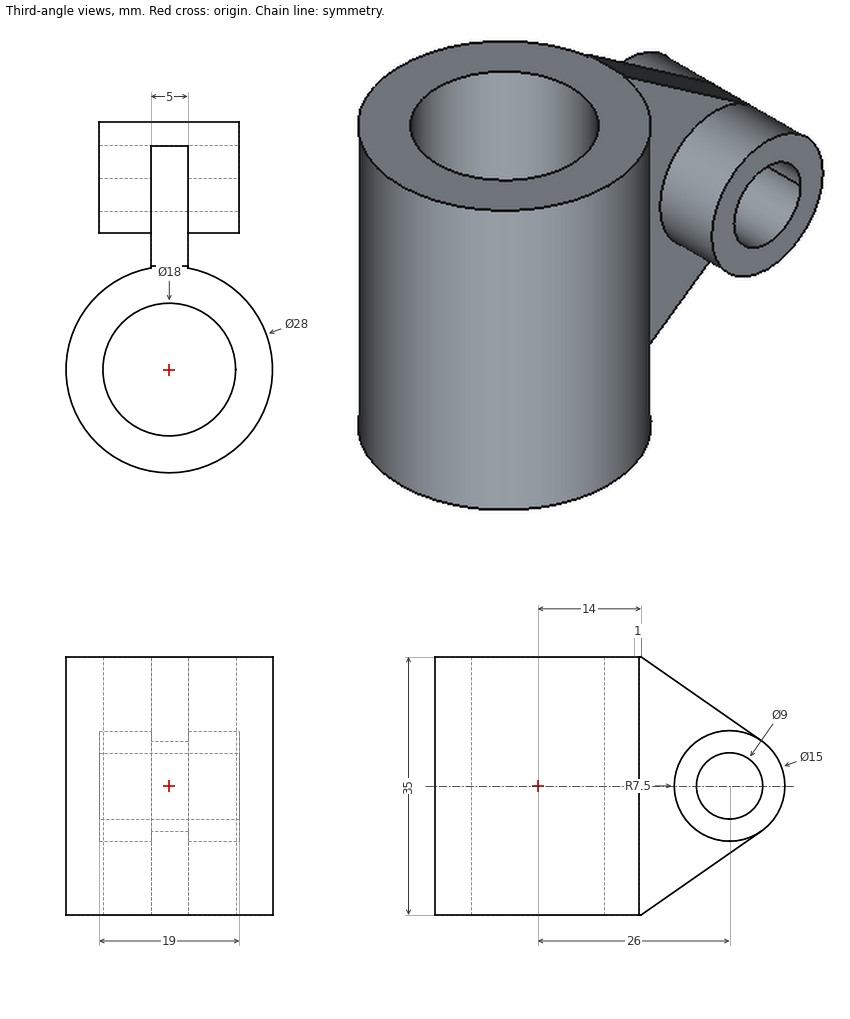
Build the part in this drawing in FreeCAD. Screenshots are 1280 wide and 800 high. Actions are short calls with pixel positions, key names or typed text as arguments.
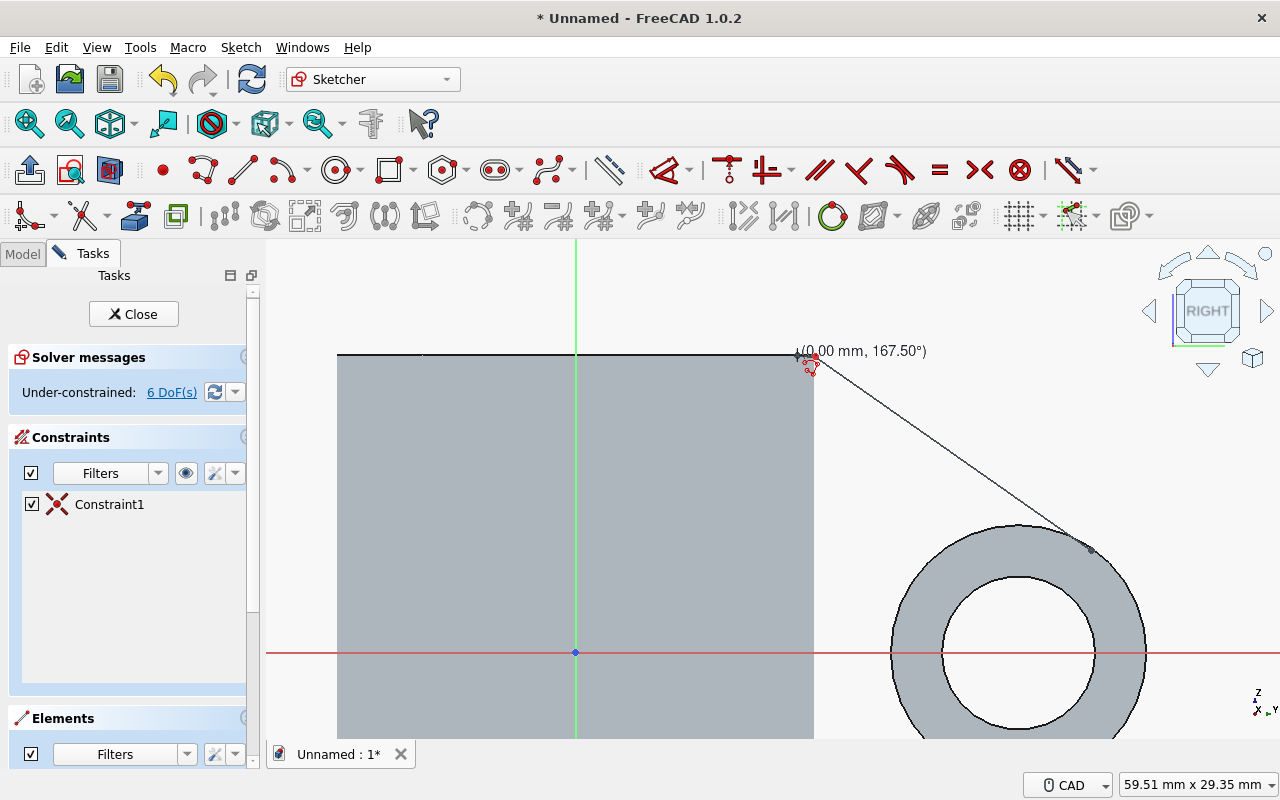
scroll(547, 290, down, 3)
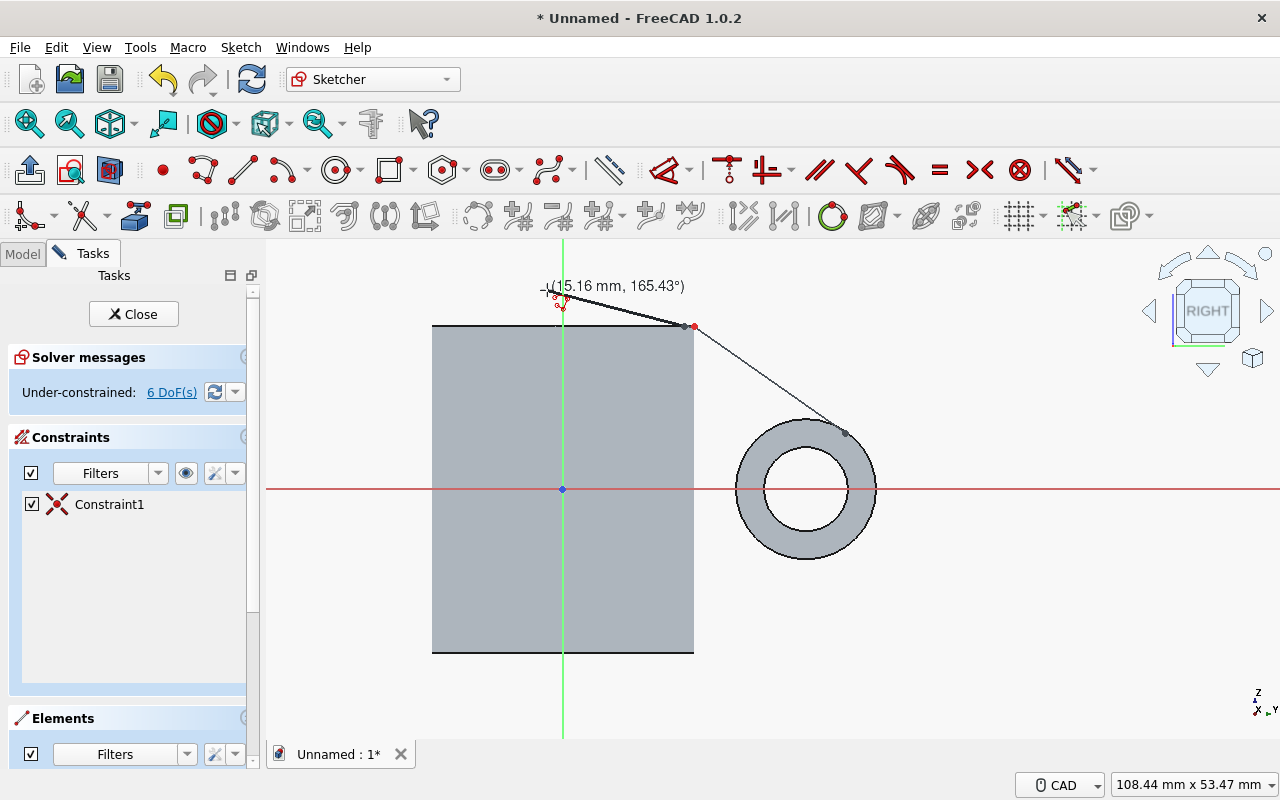
click(684, 653)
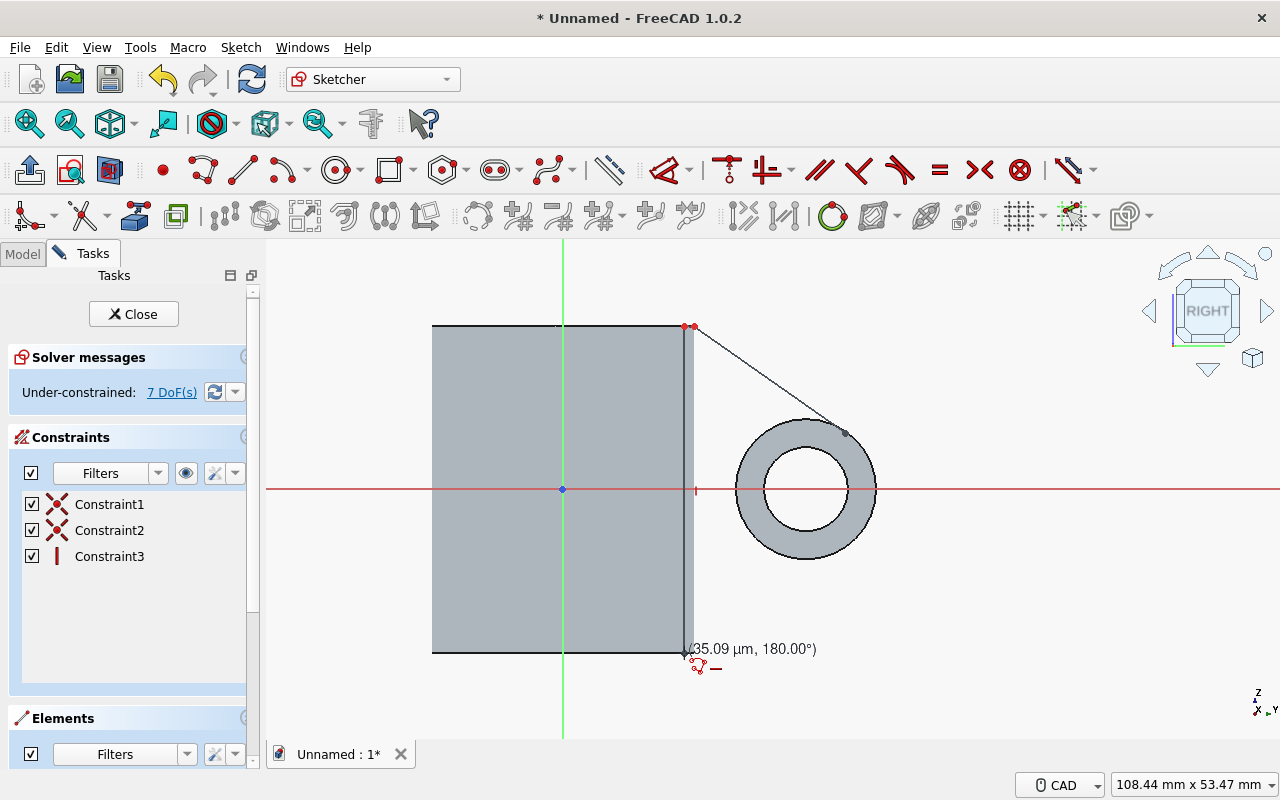
scroll(694, 653, up, 3)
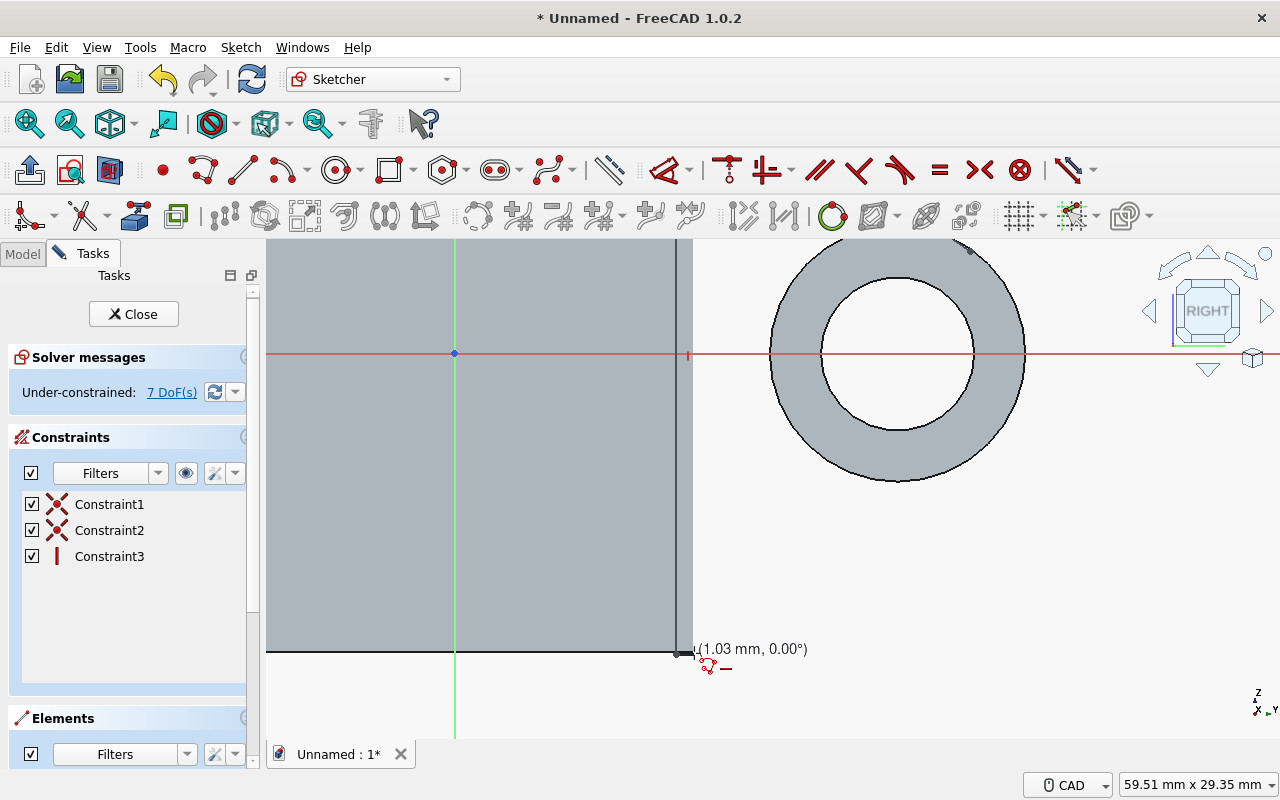
click(693, 652)
click(971, 459)
right_click(971, 459)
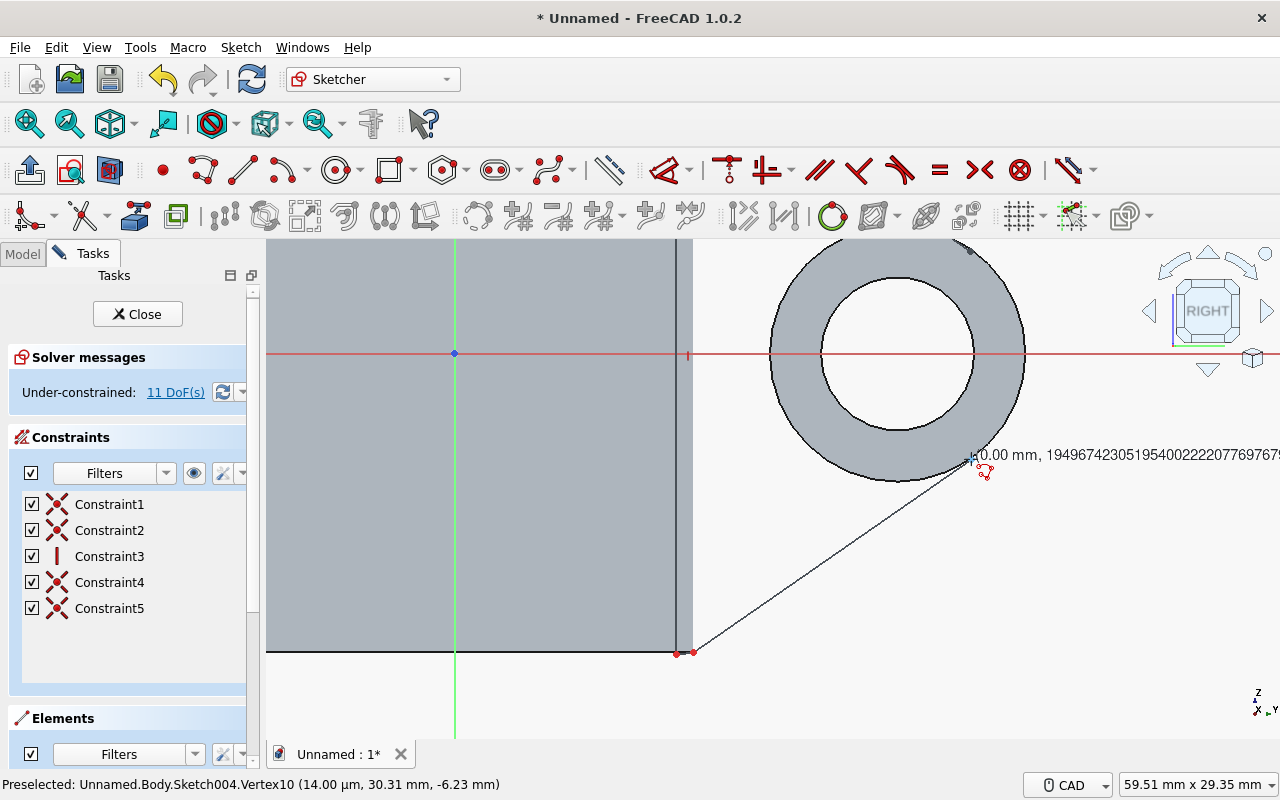
click(310, 170)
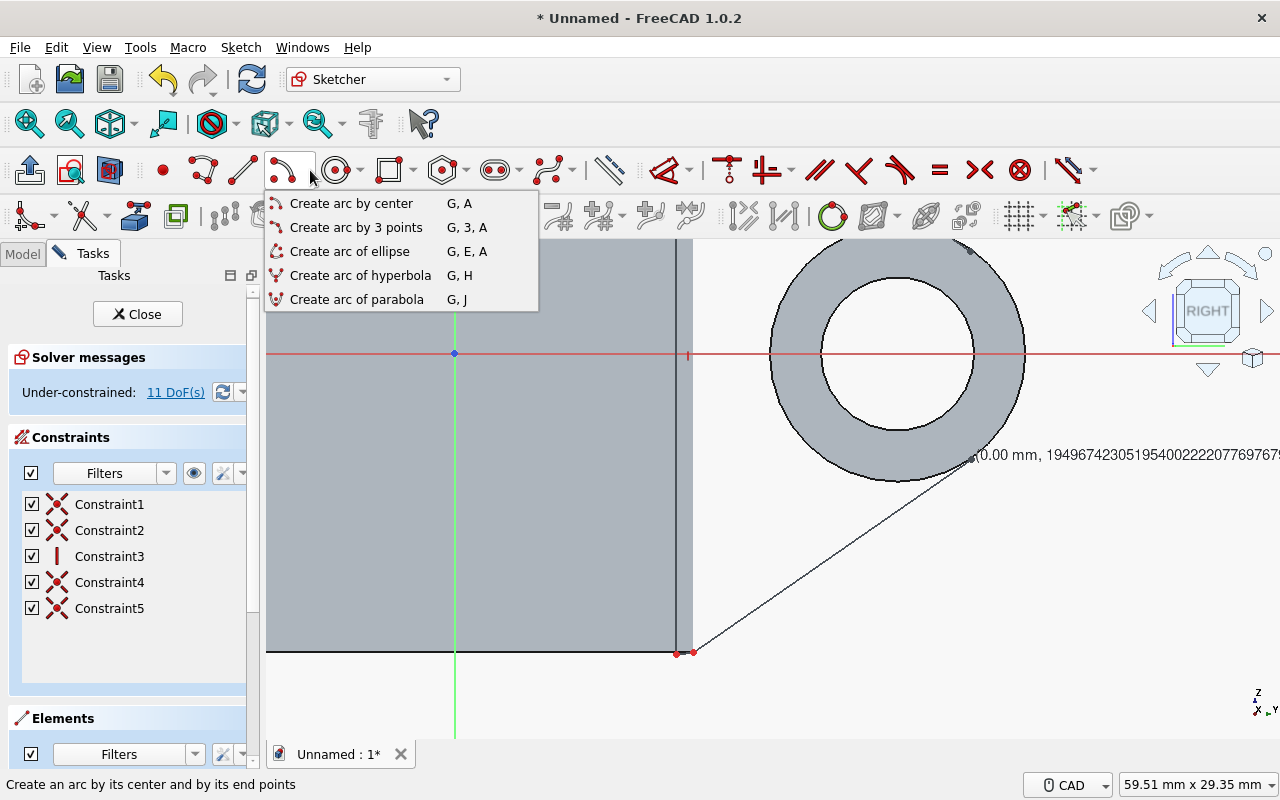
click(402, 227)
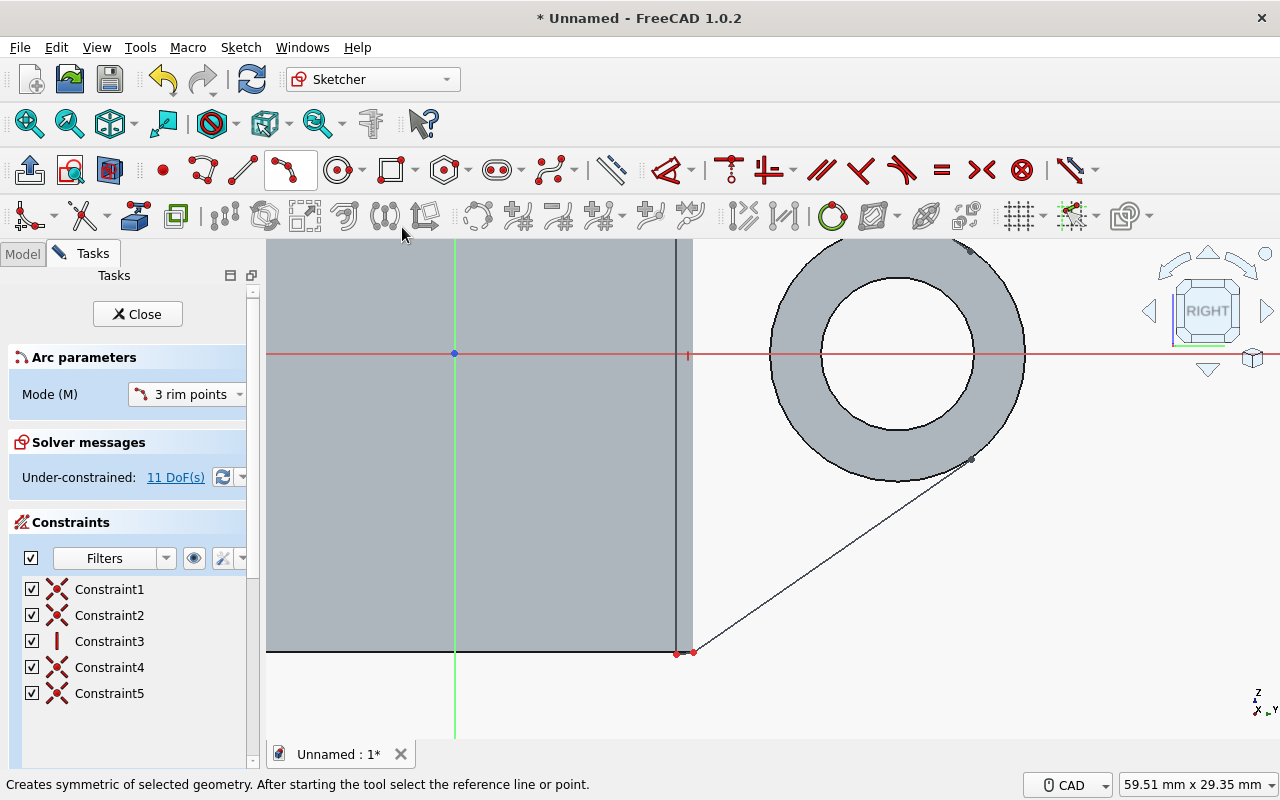
click(971, 460)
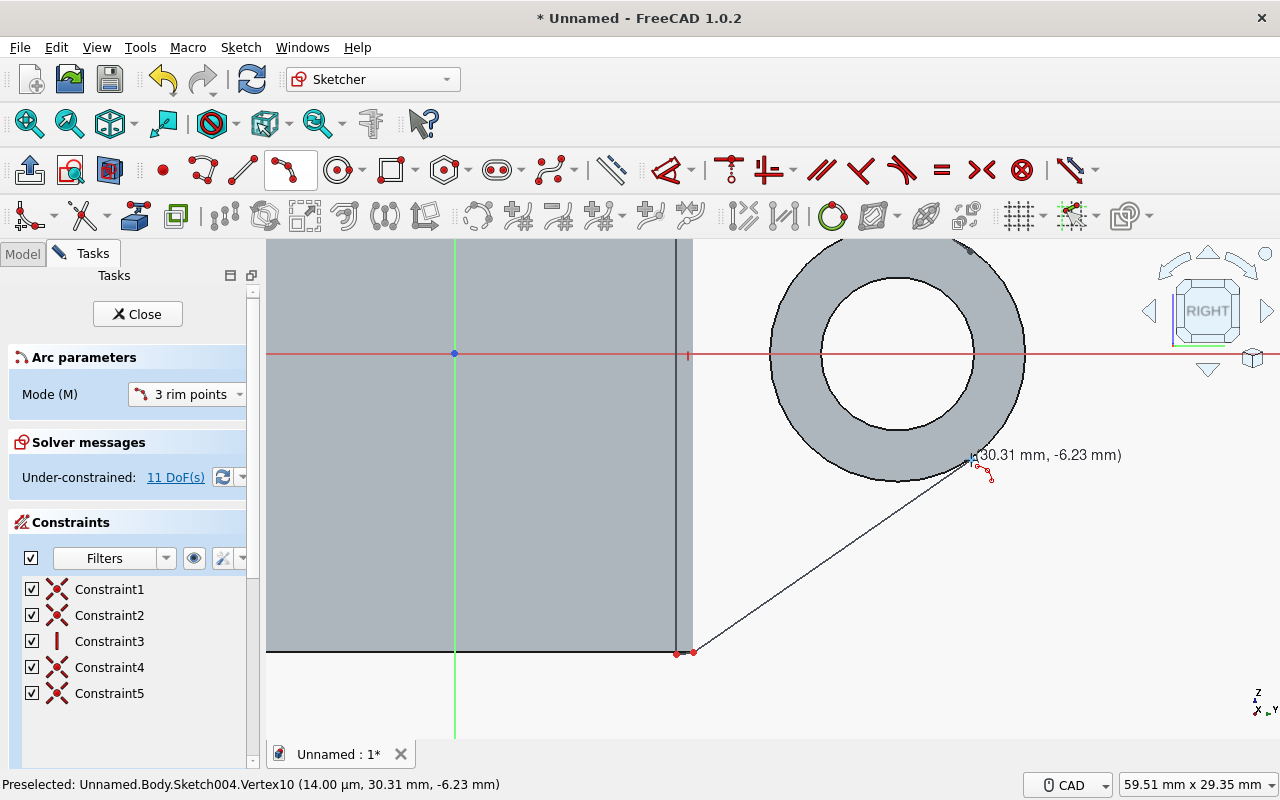
scroll(695, 653, down, 3)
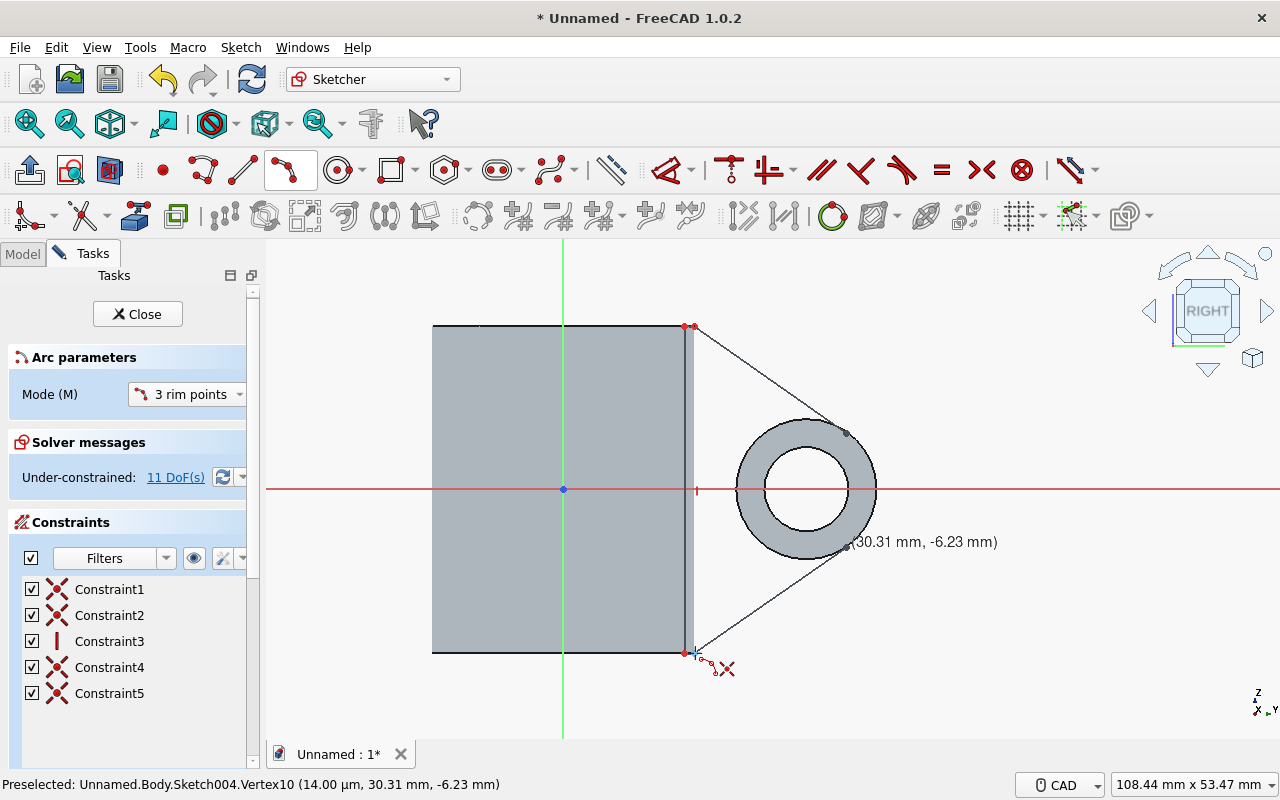
click(846, 433)
click(743, 460)
key(Escape)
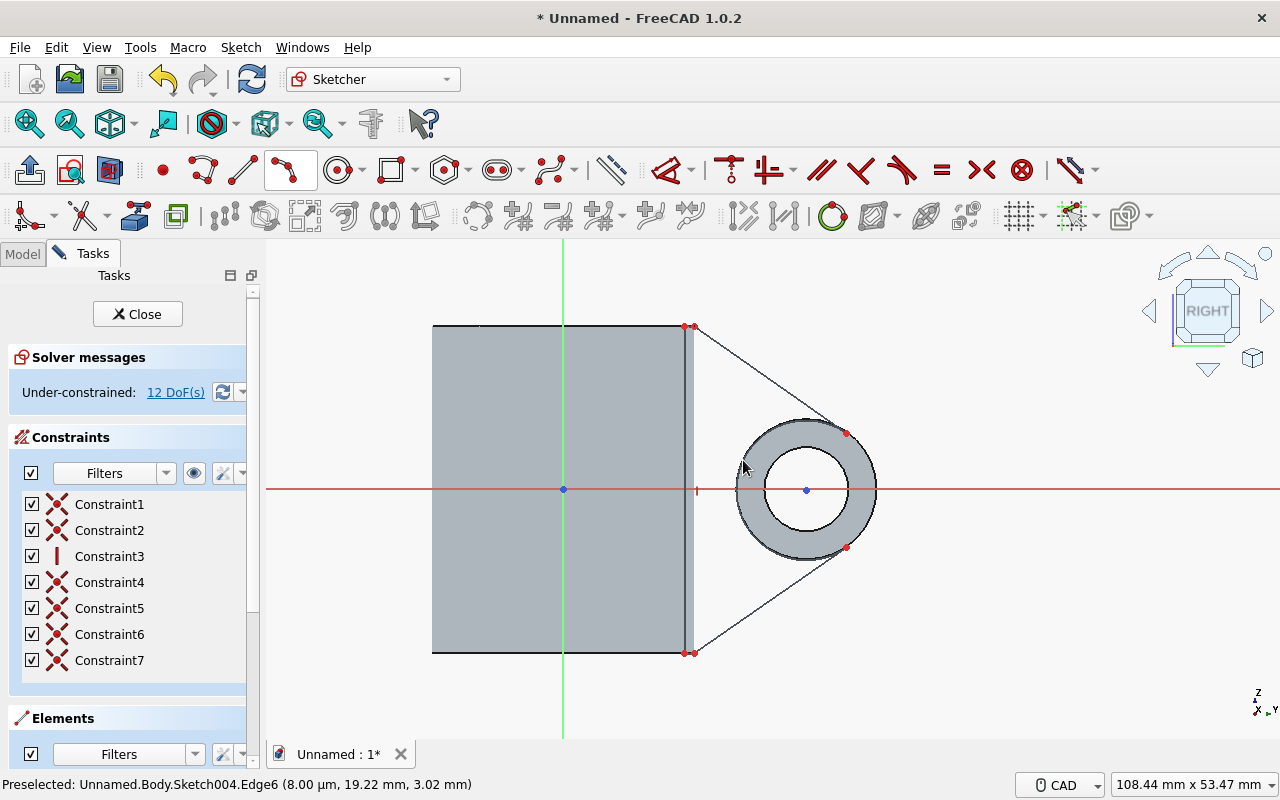
click(801, 401)